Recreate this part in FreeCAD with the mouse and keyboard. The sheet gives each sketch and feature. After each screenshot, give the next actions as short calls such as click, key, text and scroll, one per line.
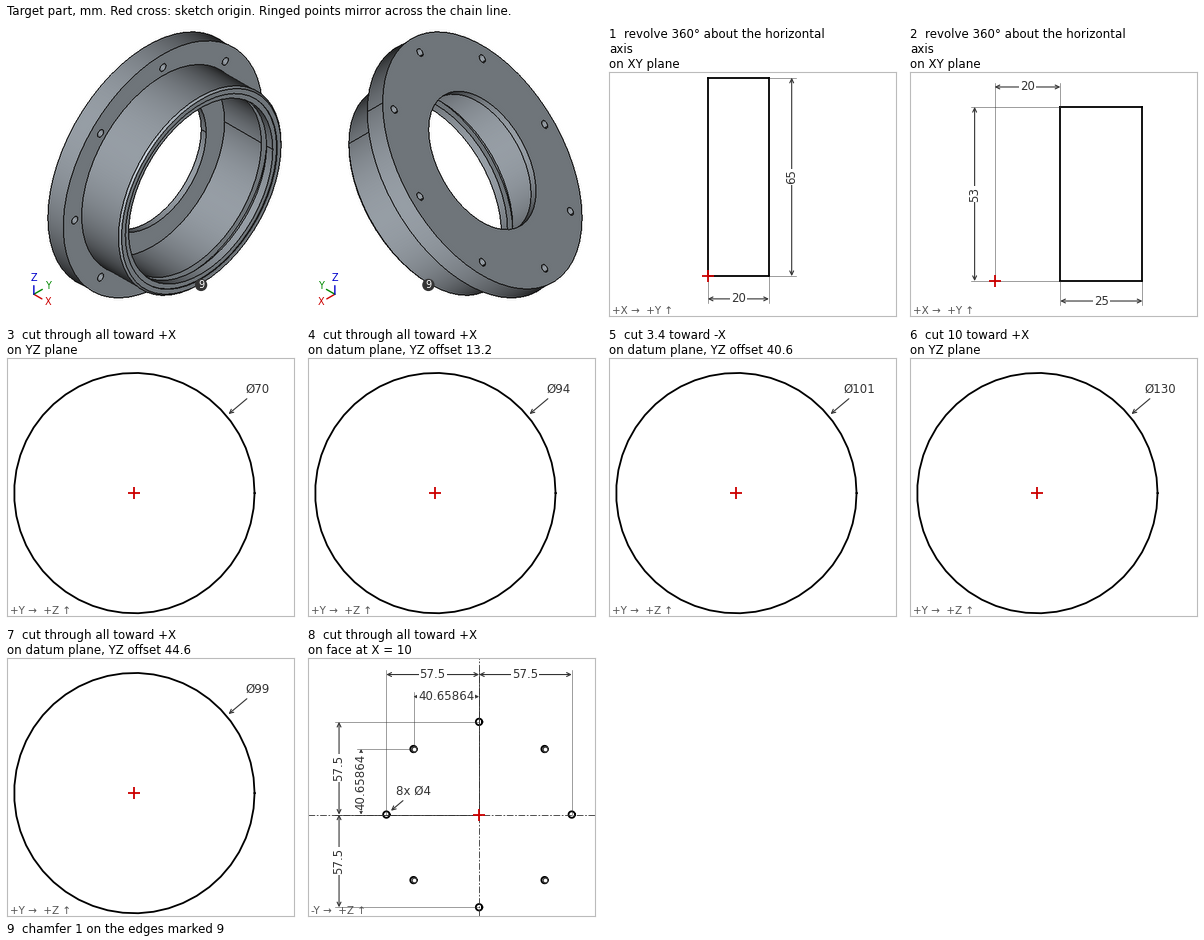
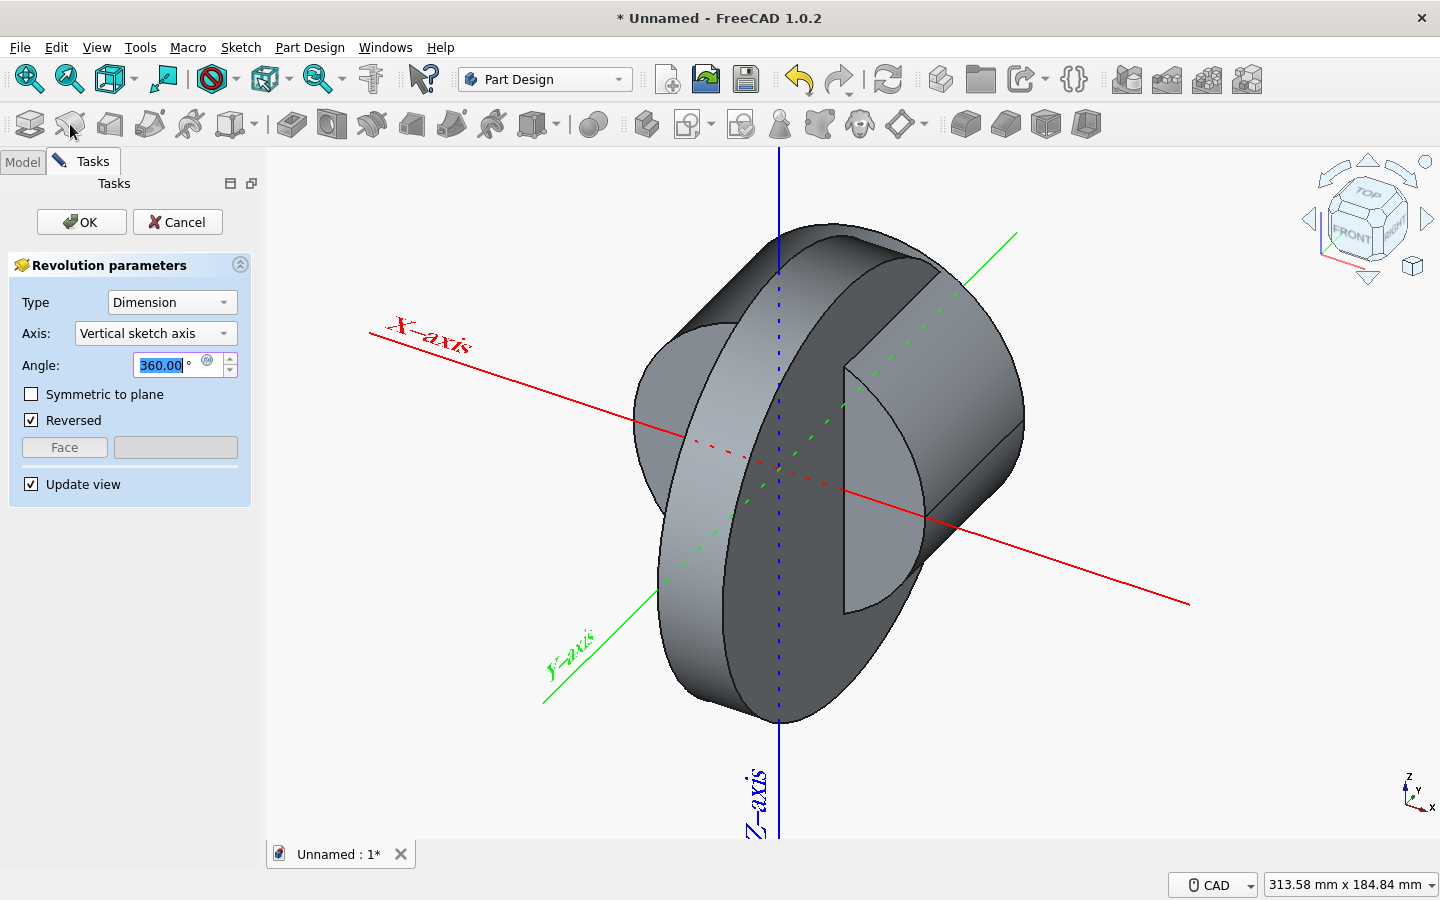
click(156, 334)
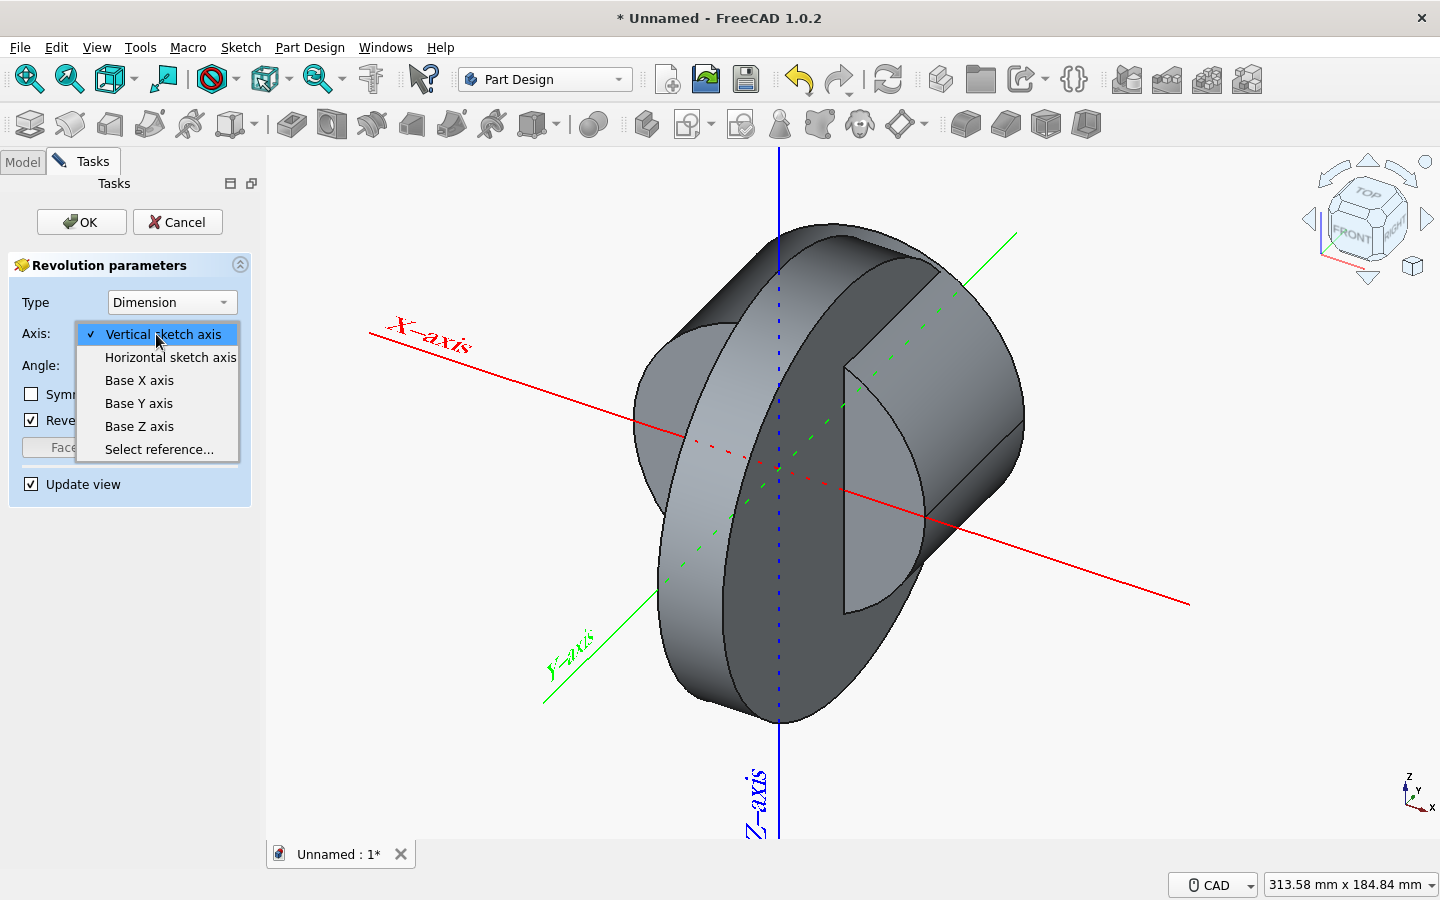
click(156, 358)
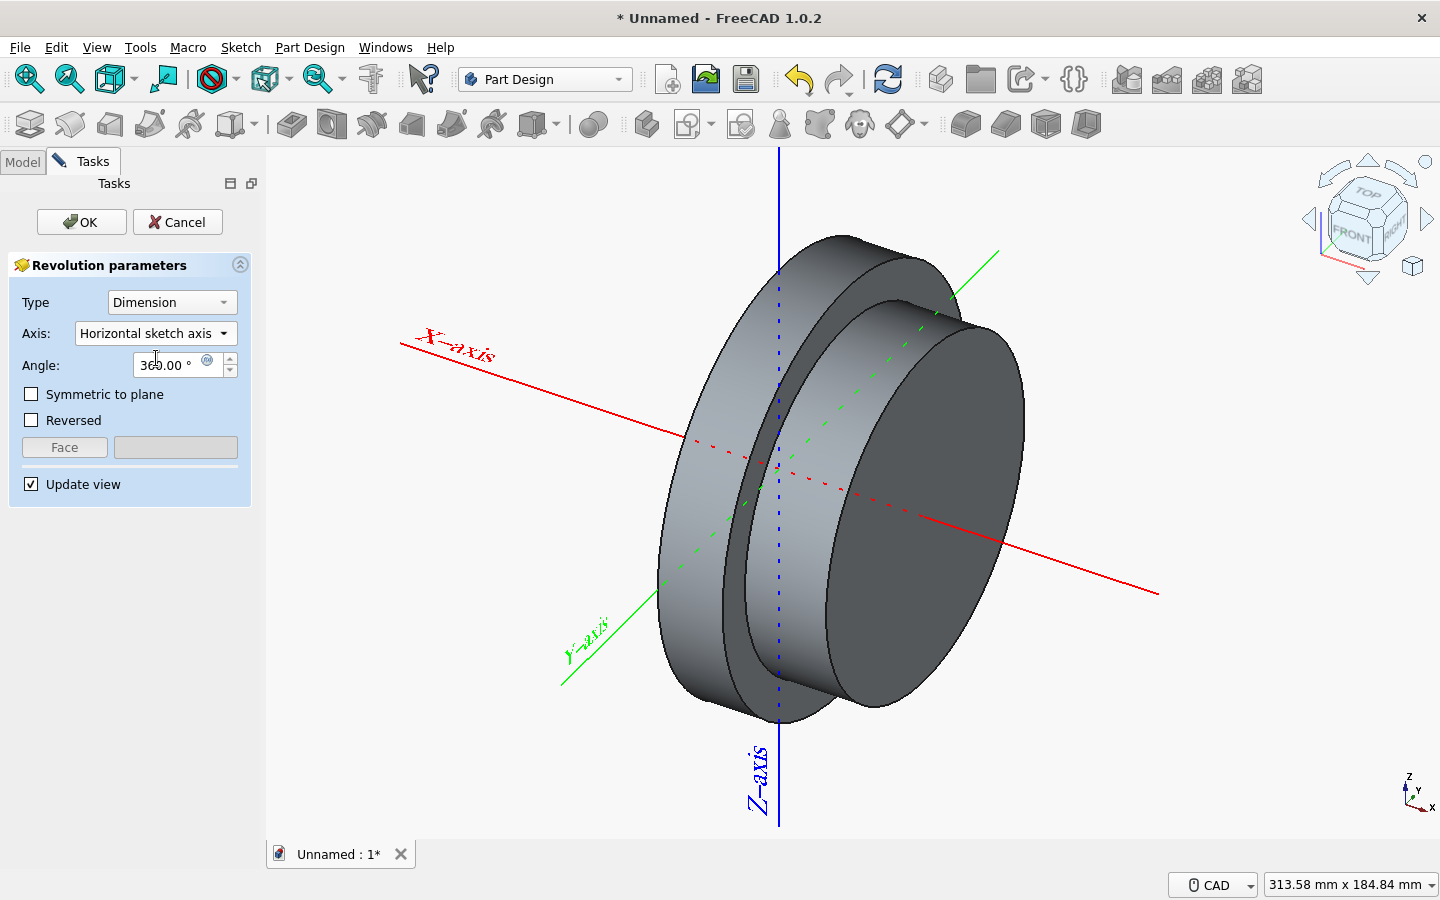
click(82, 222)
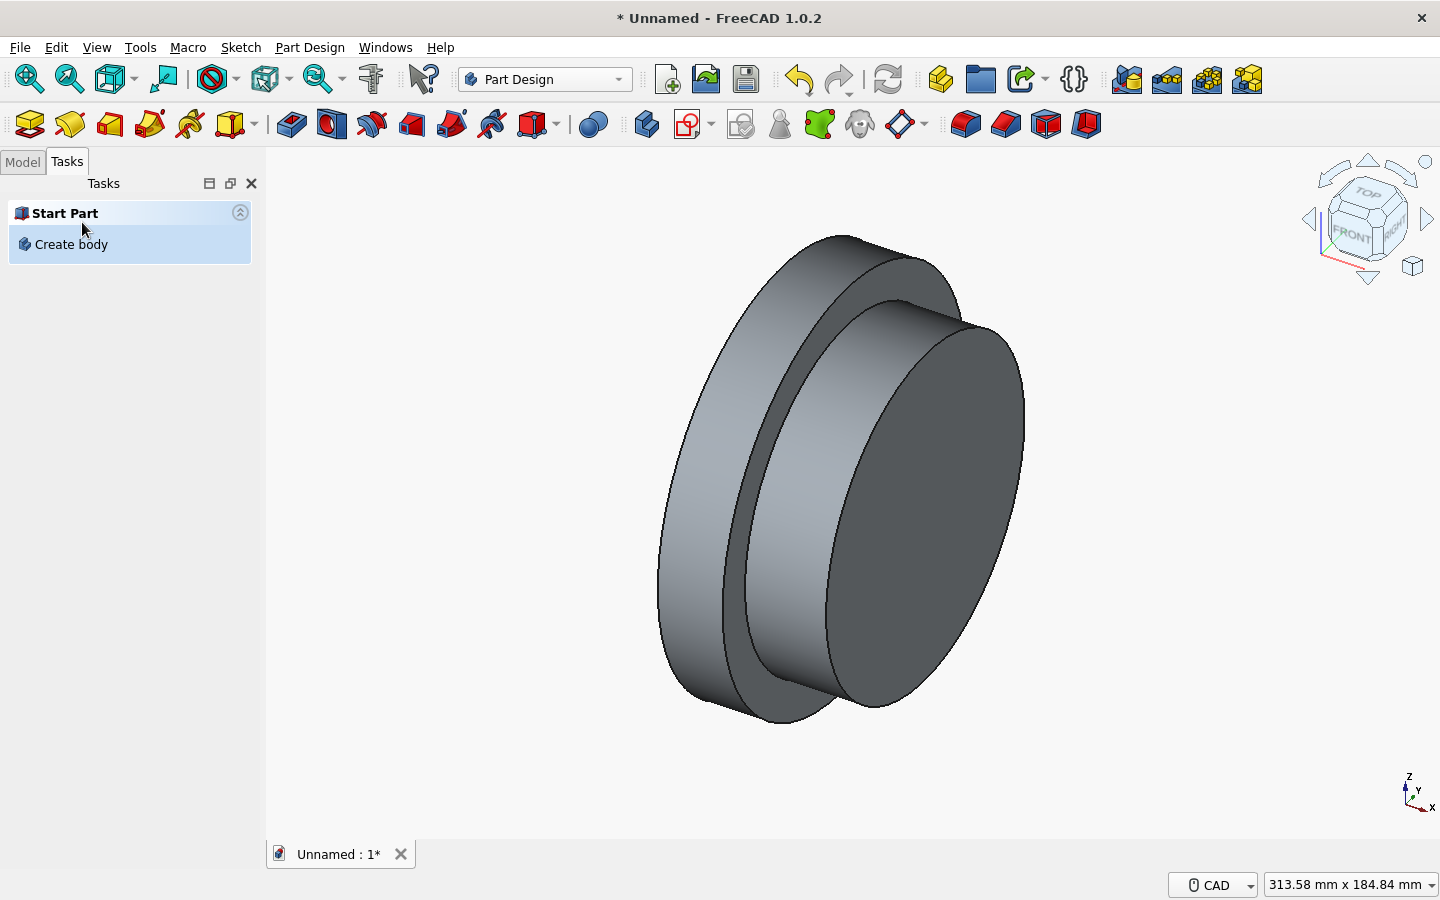
click(688, 124)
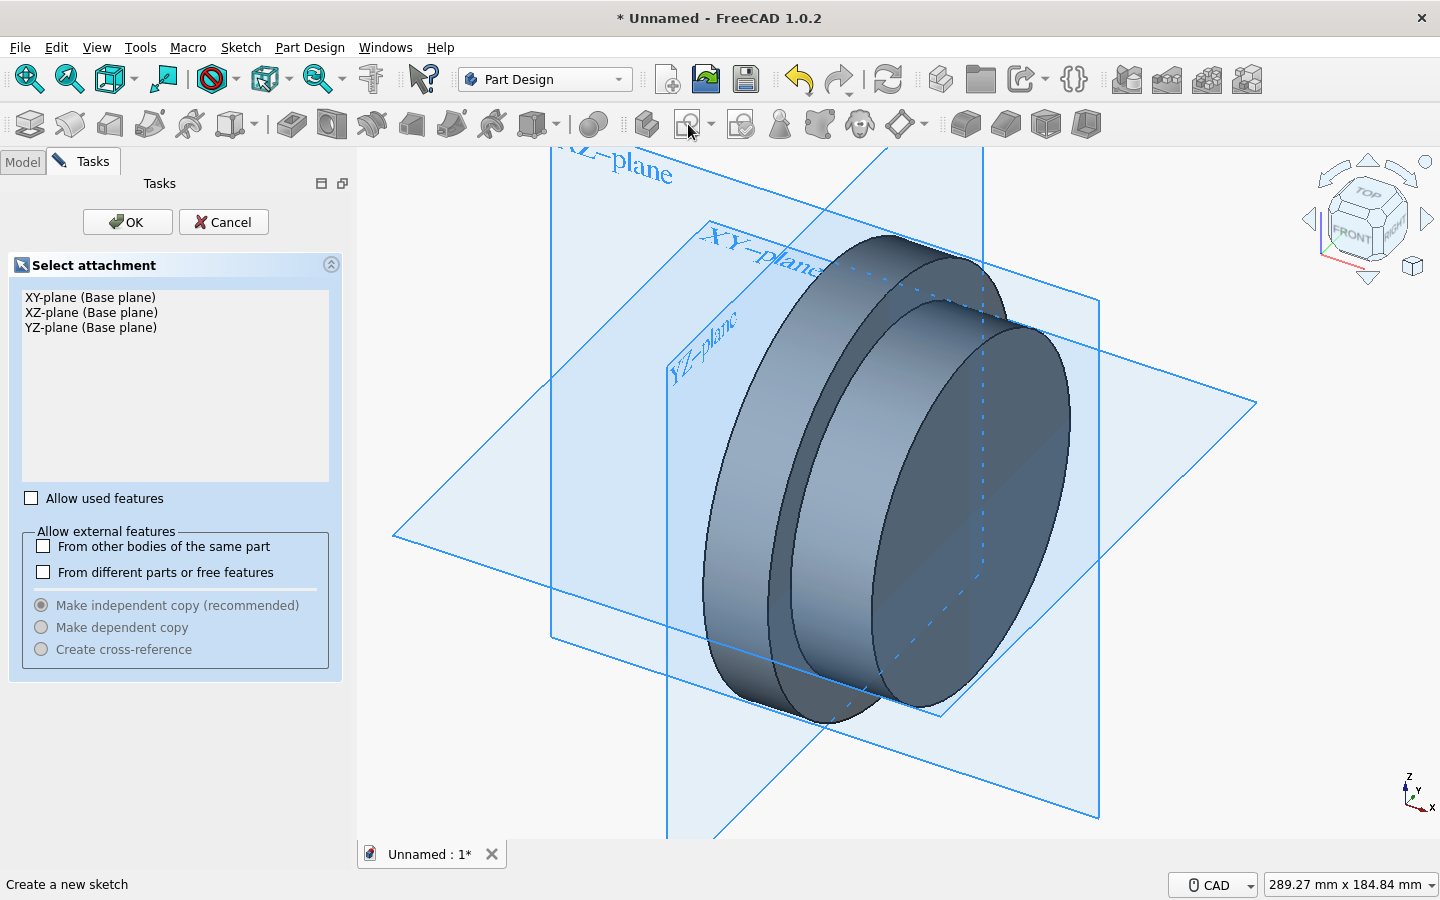
click(82, 328)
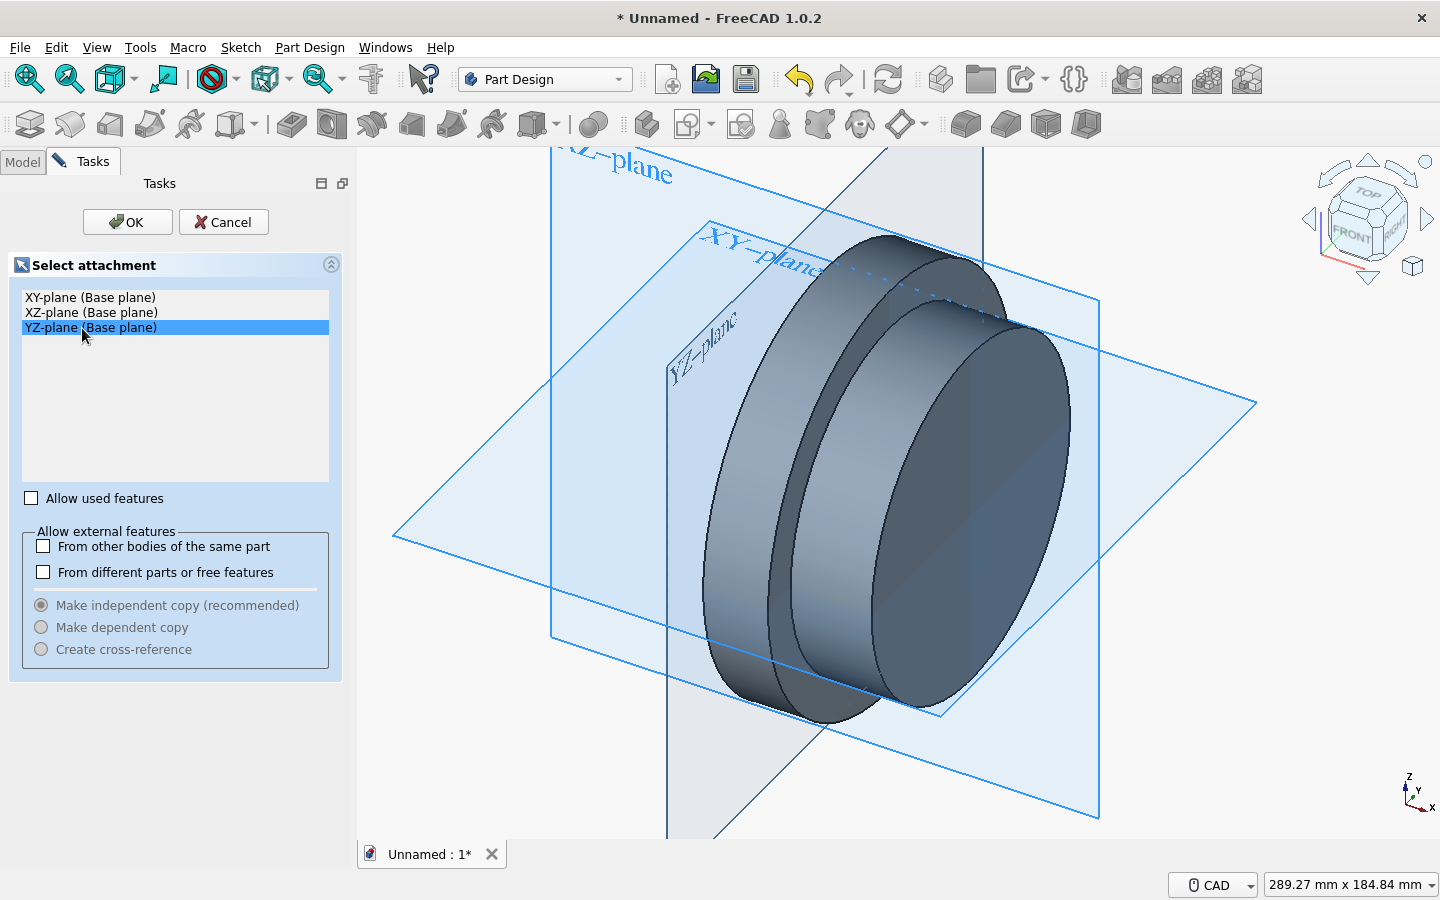
click(128, 222)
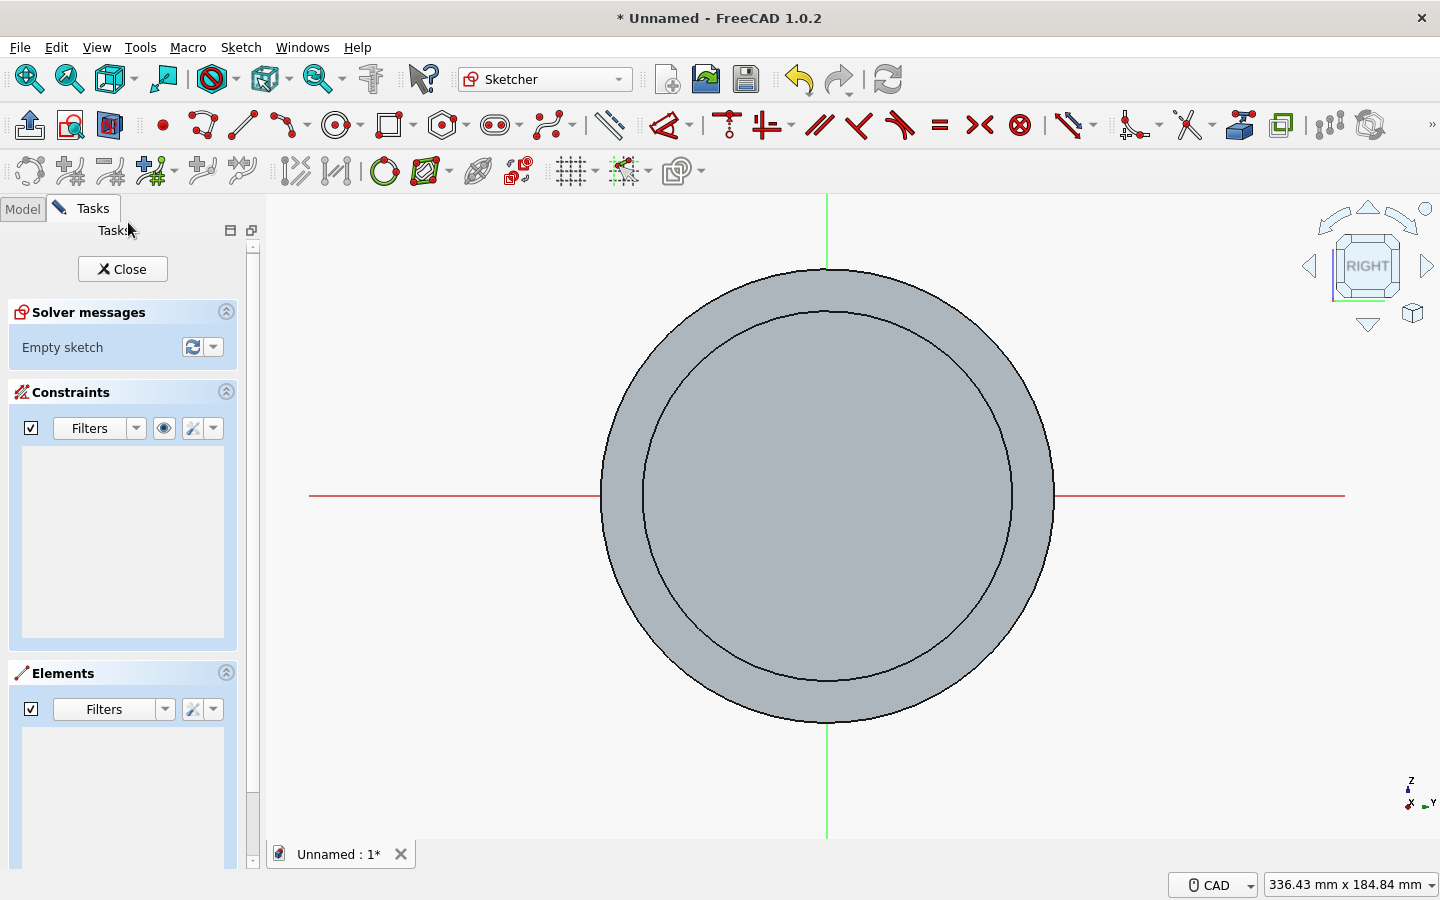
click(110, 126)